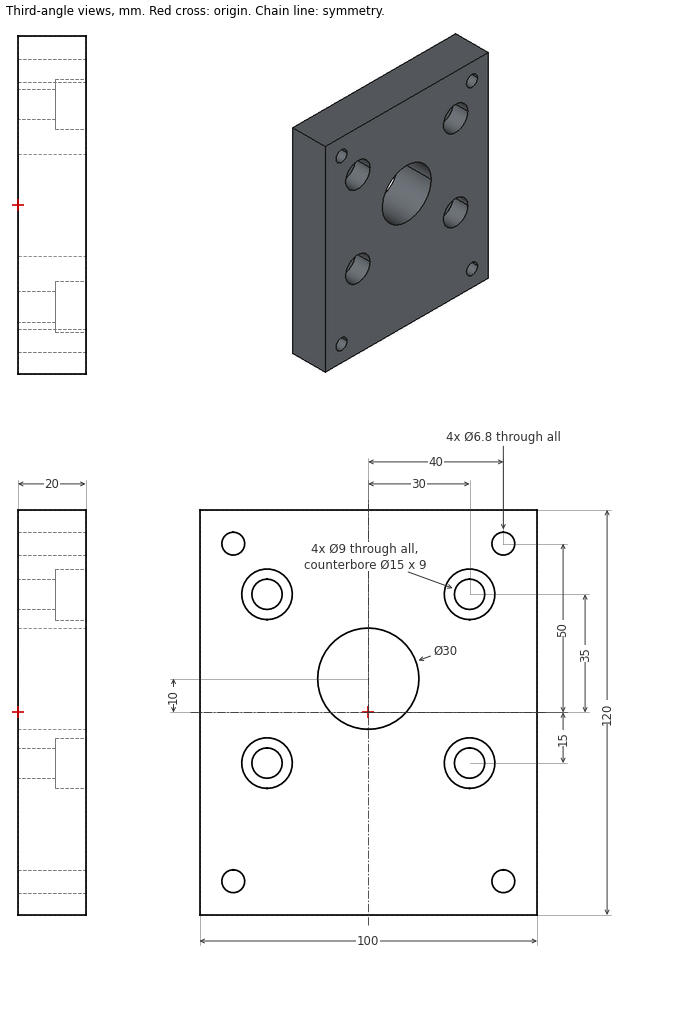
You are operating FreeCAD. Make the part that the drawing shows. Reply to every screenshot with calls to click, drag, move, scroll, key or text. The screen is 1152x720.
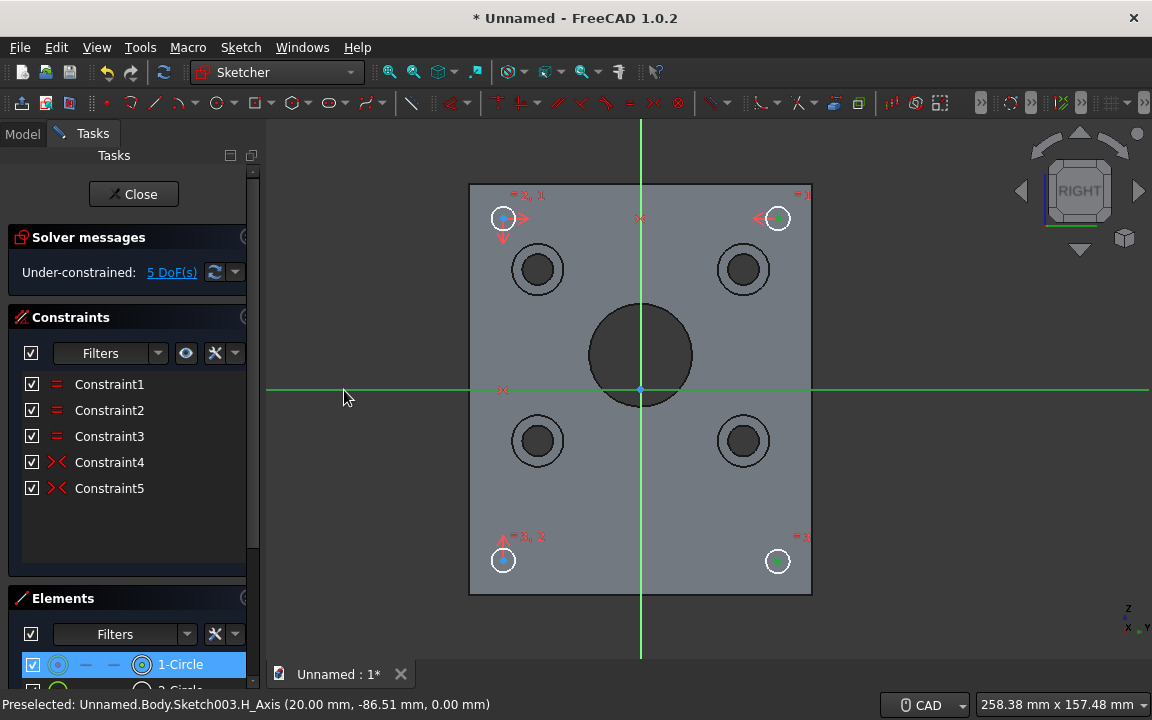
click(654, 104)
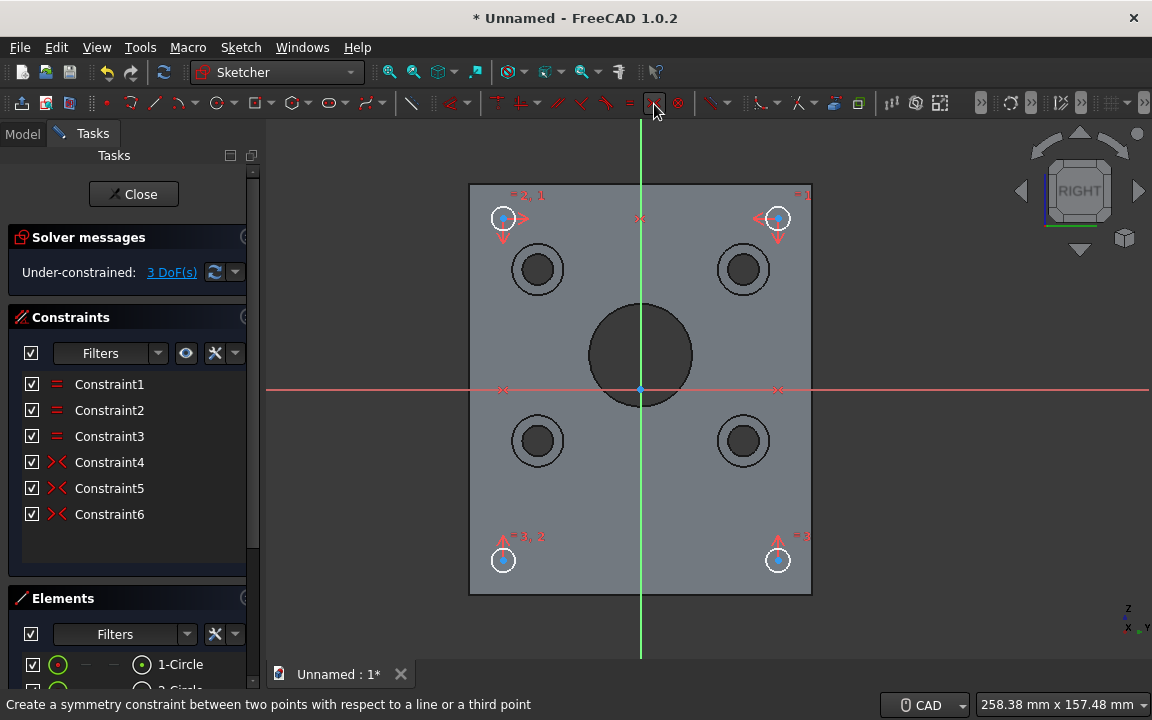
click(450, 104)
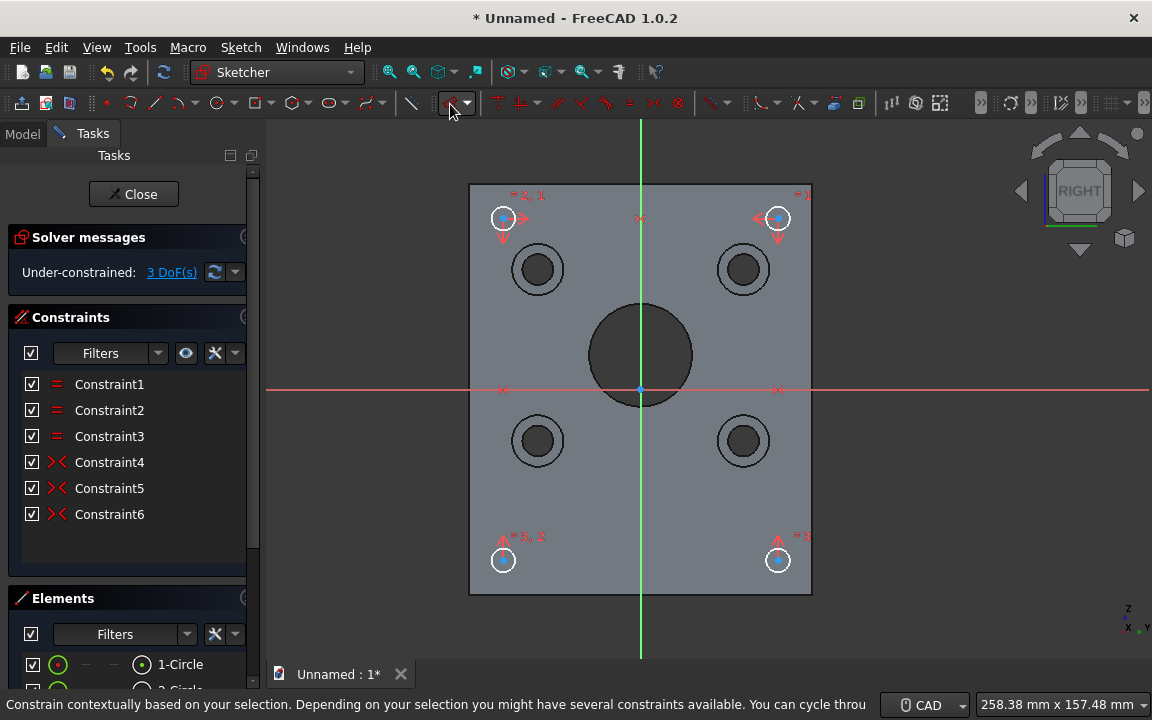
scroll(786, 210, up, 3)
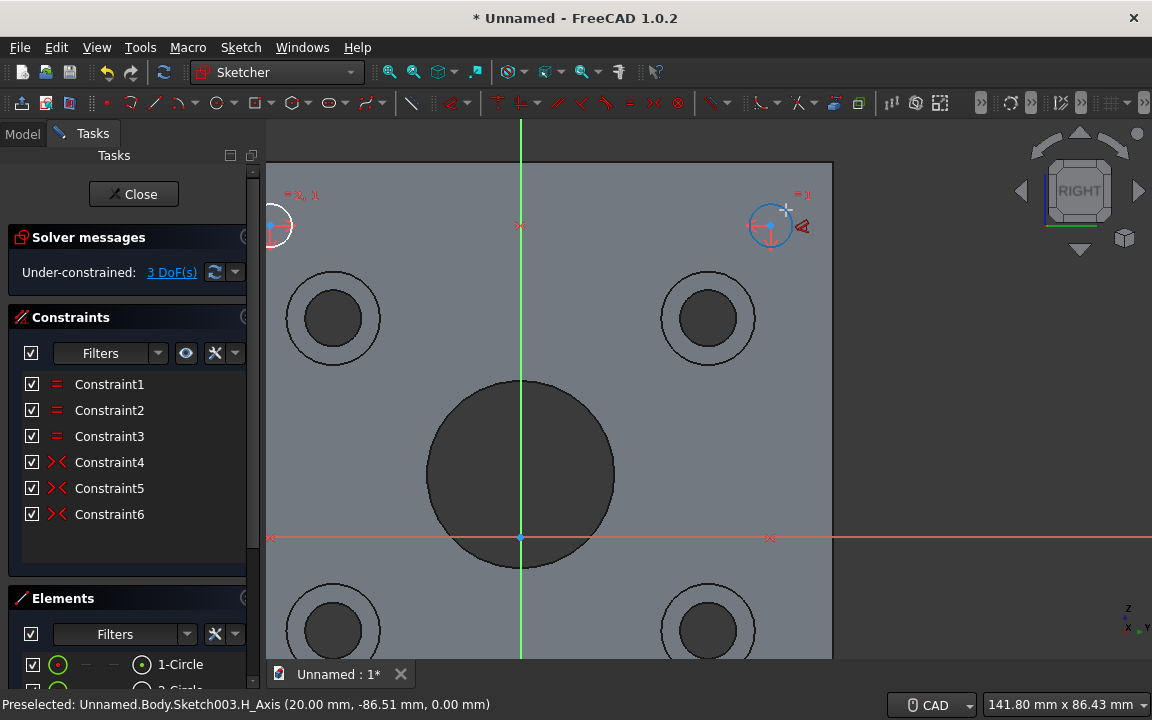
click(786, 210)
click(808, 187)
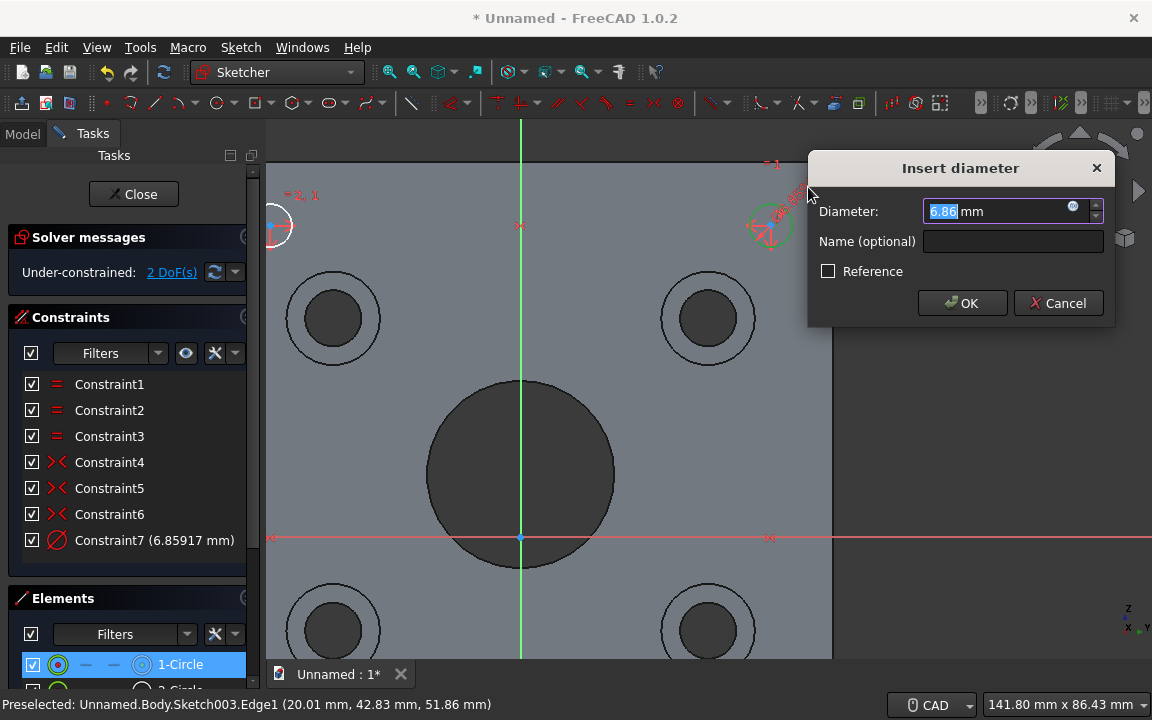
text(6.8)
key(Return)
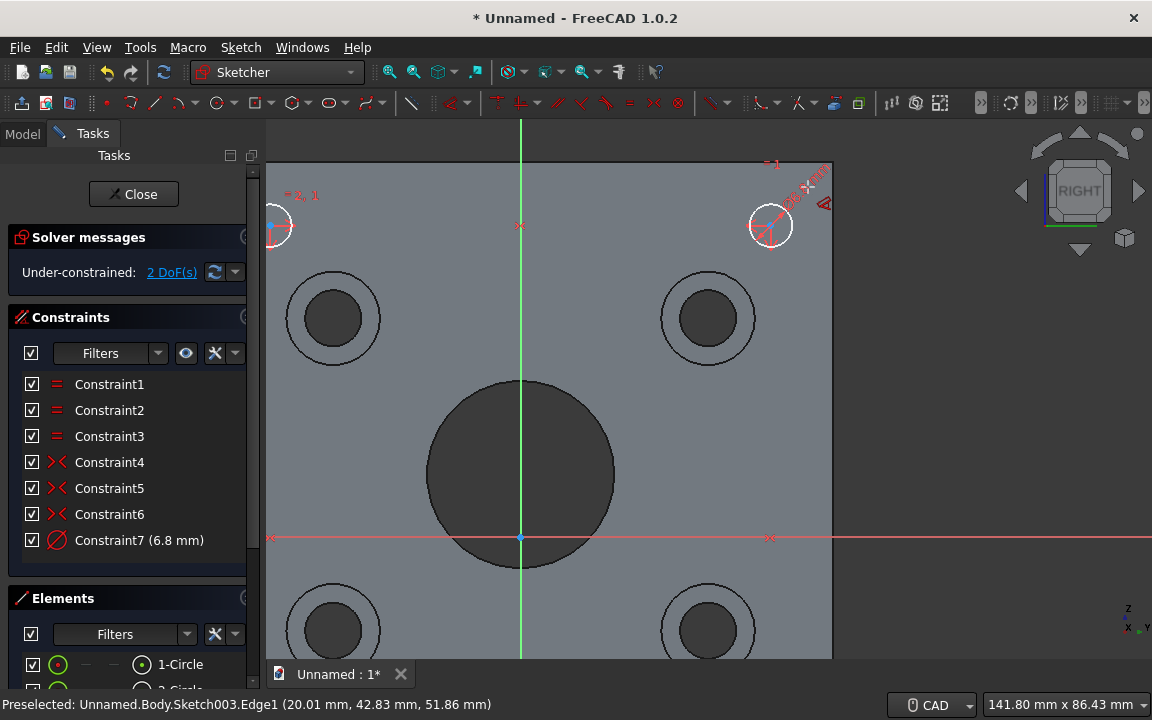
click(771, 226)
click(646, 192)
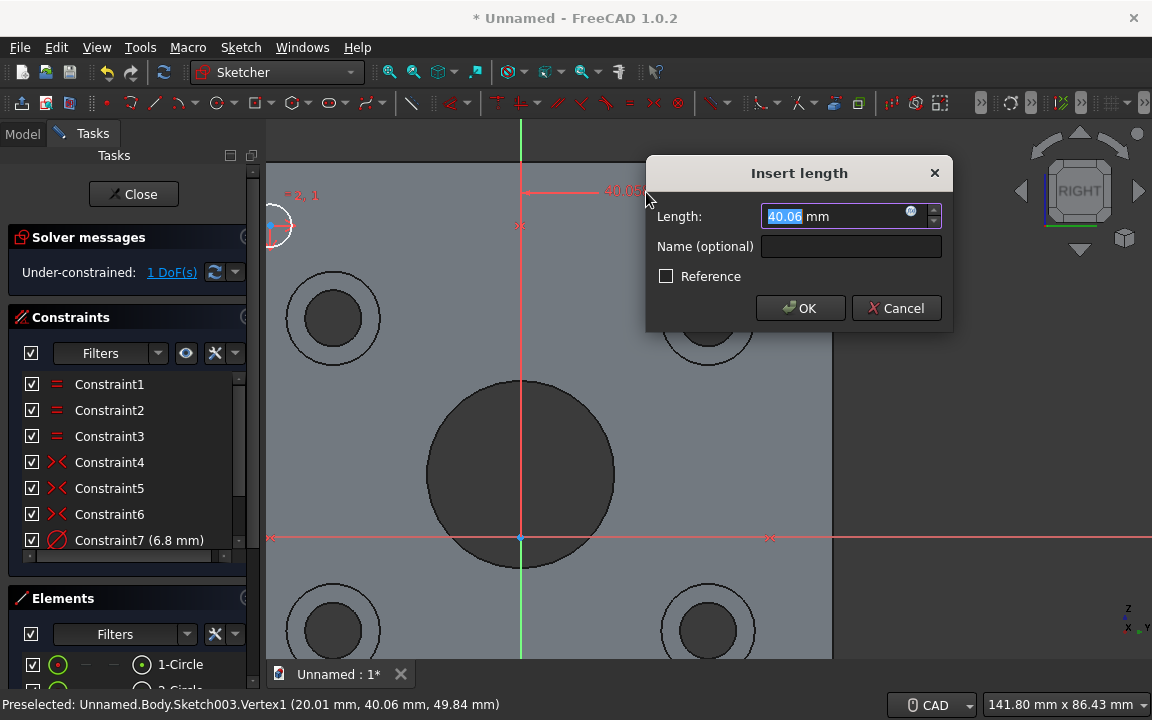
text(40)
key(Return)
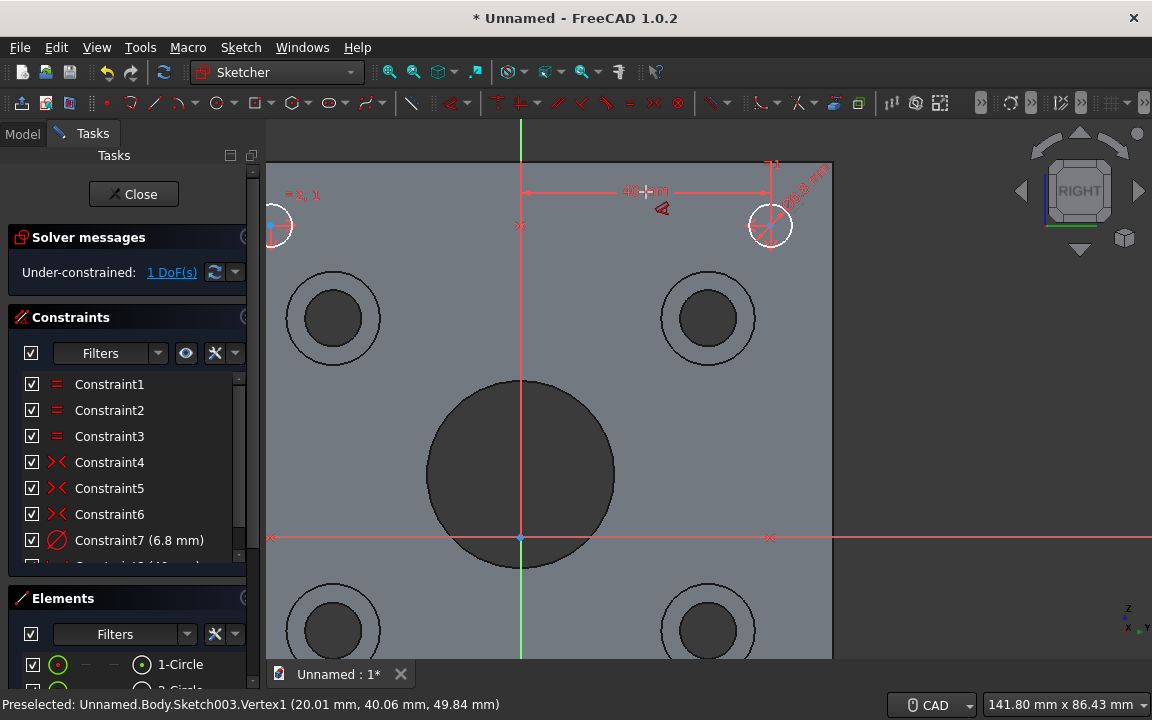
click(771, 226)
click(805, 381)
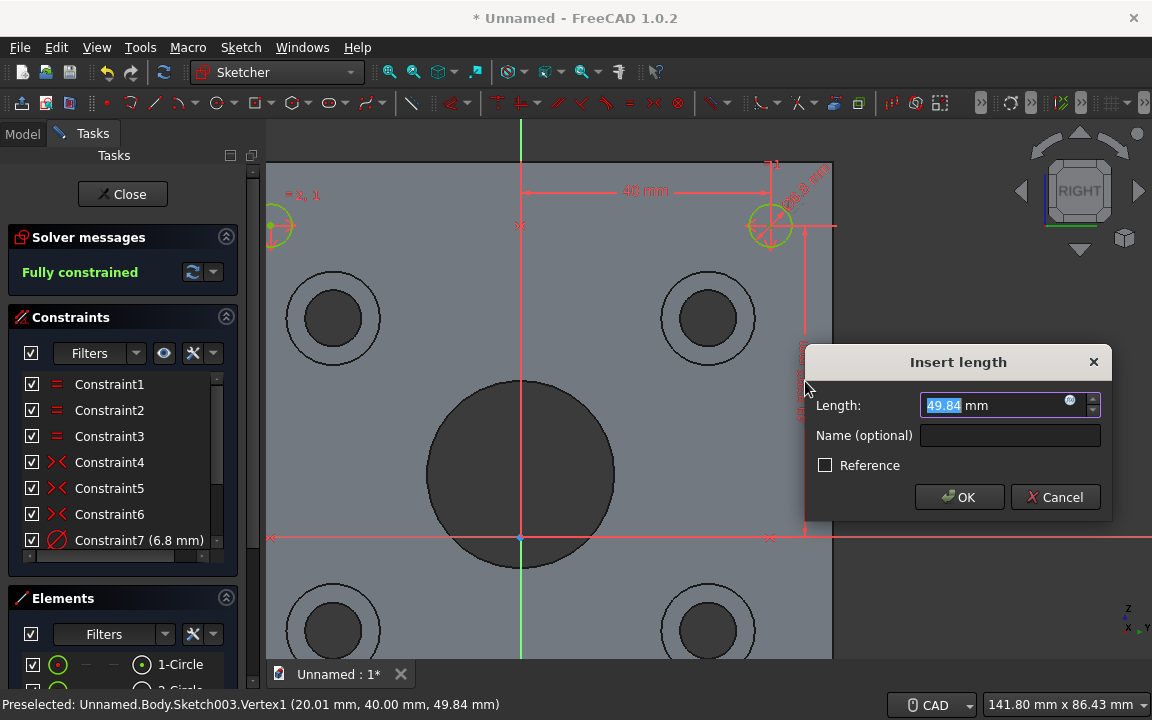
text(50)
key(Return)
key(Escape)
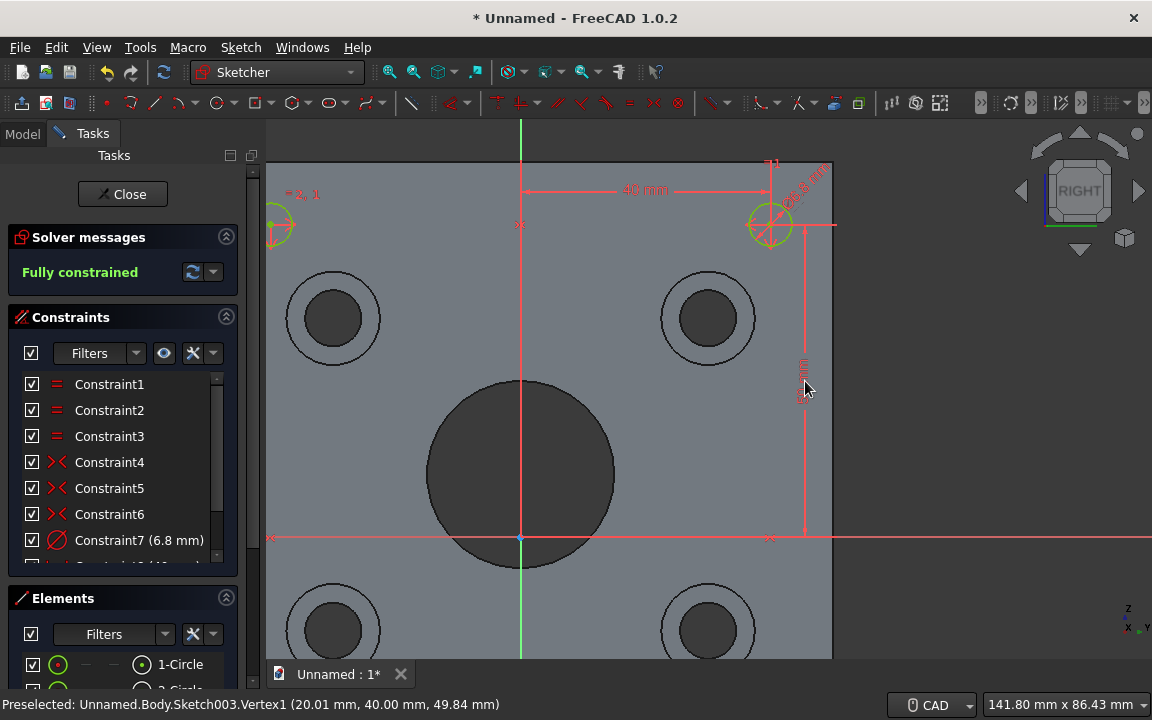
click(123, 194)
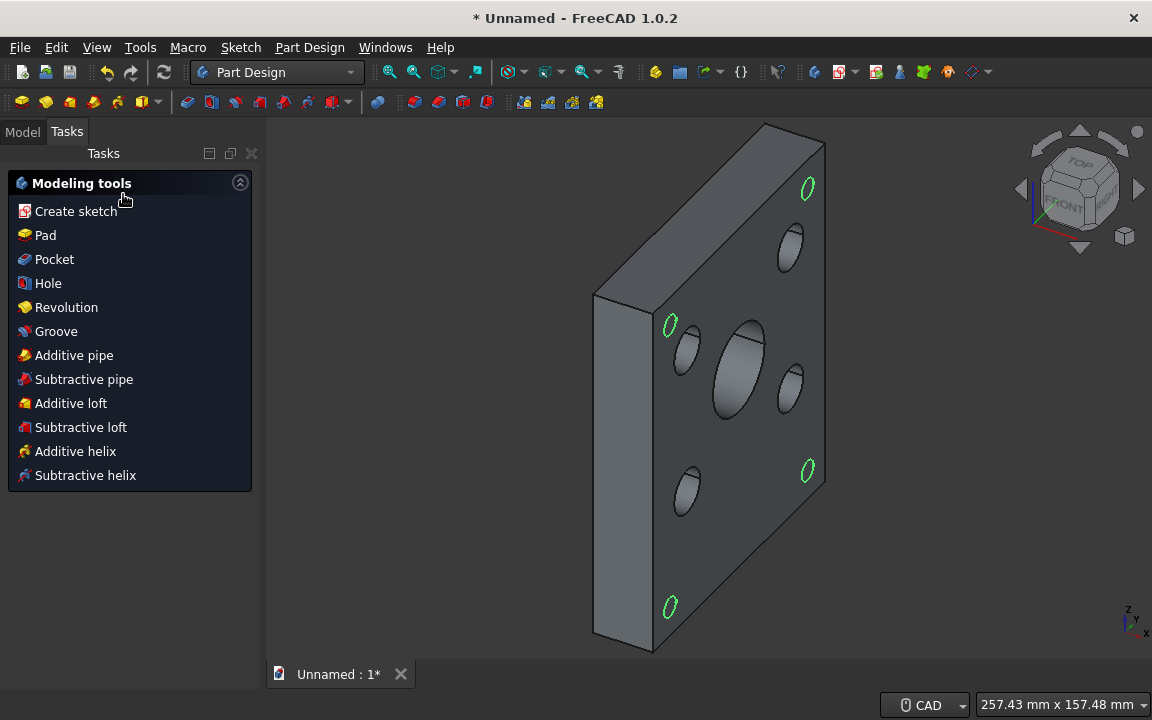
click(212, 102)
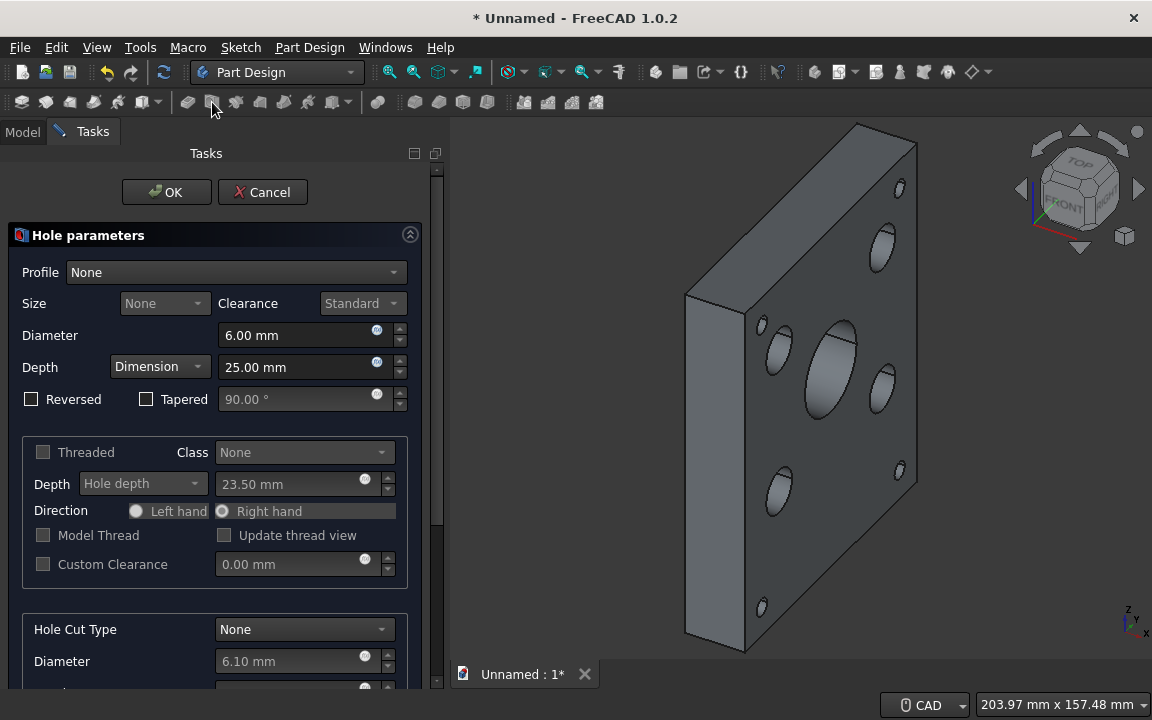
triple_click(305, 335)